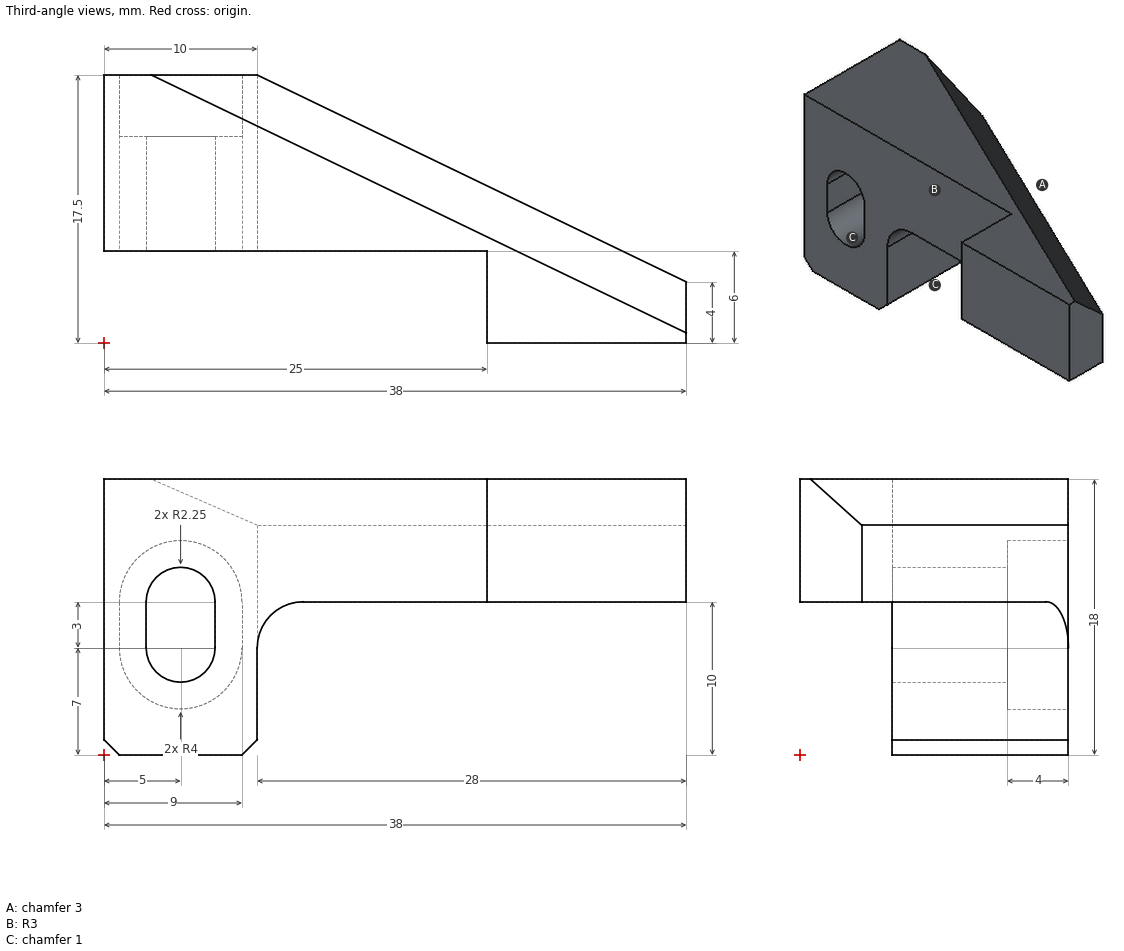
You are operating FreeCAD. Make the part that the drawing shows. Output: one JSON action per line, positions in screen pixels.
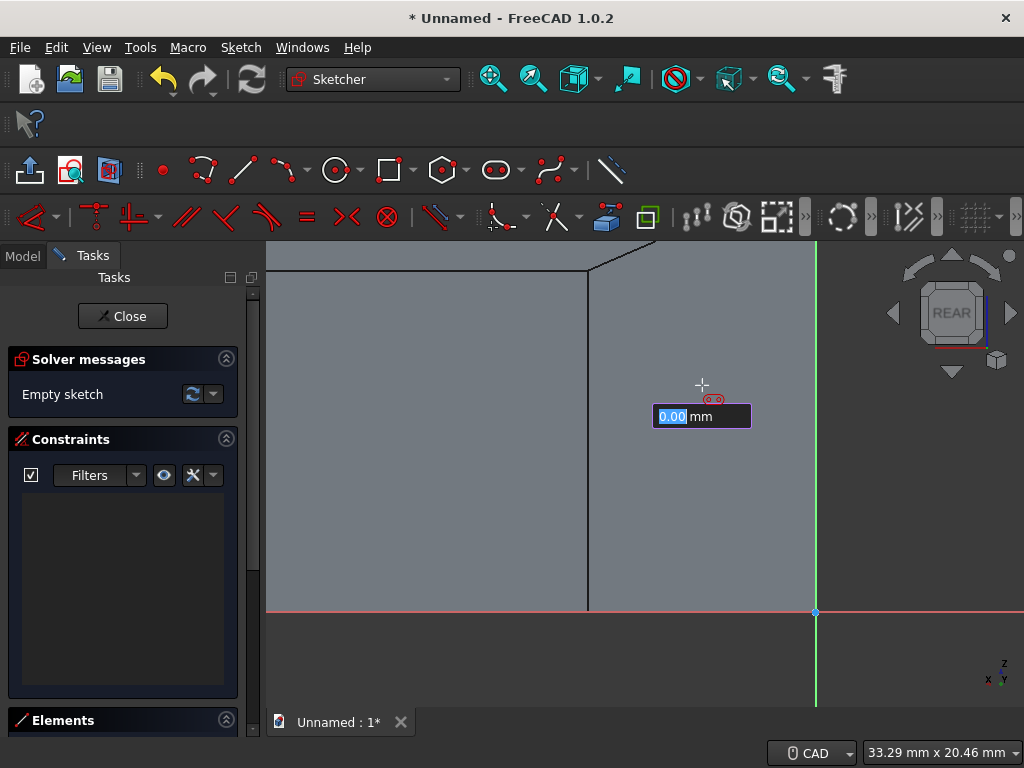
{"action": "left_click", "coordinate": [753, 419]}
{"action": "key", "text": "Escape"}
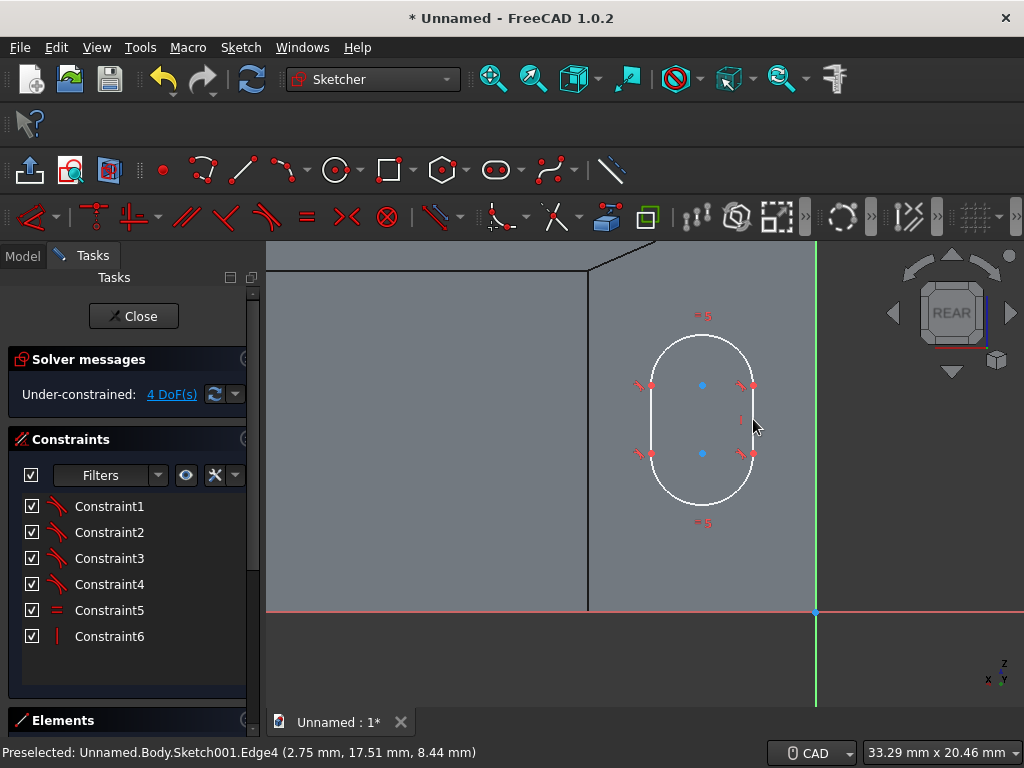
{"action": "key", "text": "d"}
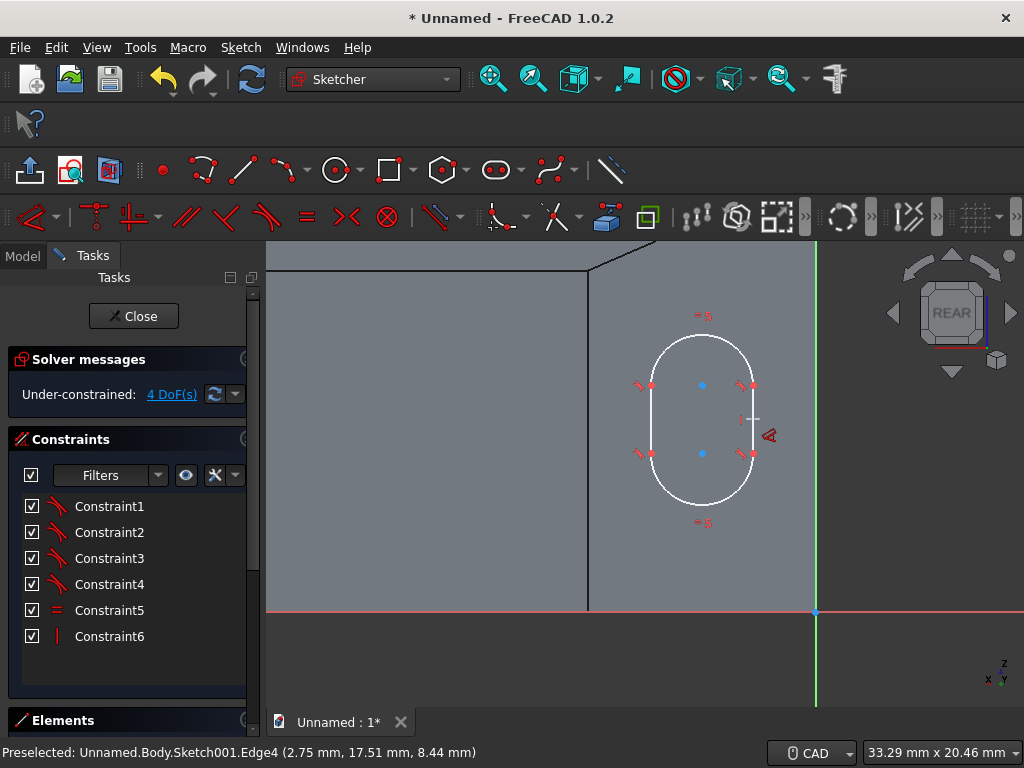
{"action": "left_click", "coordinate": [672, 495]}
{"action": "left_click", "coordinate": [653, 521]}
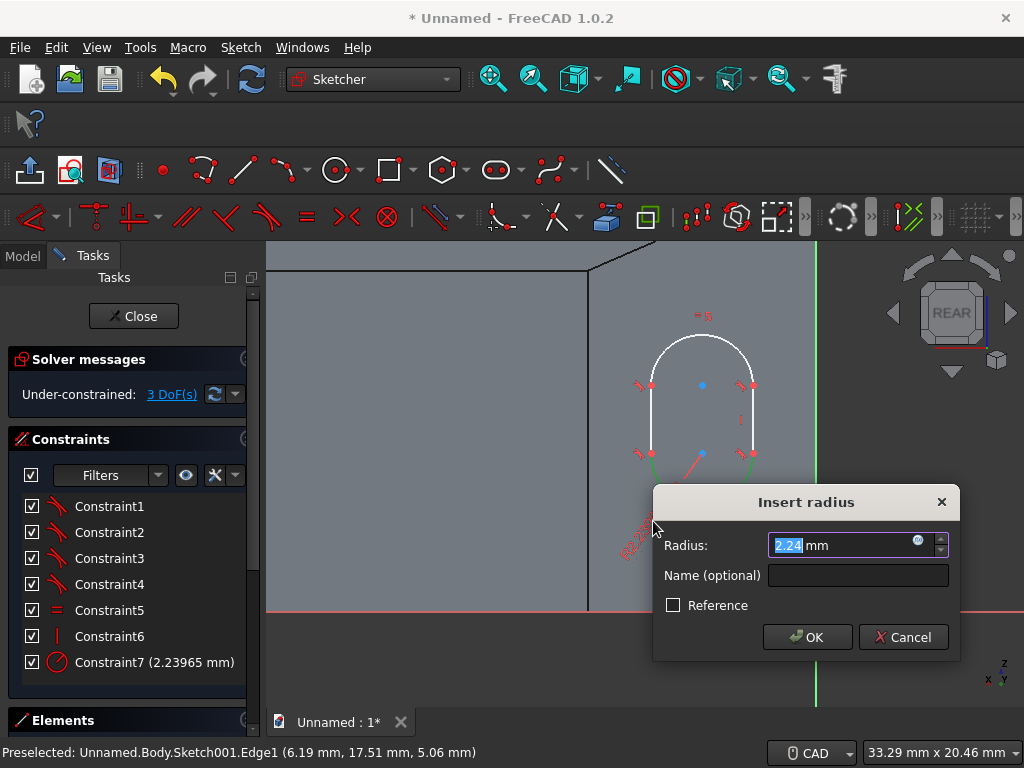
{"action": "type", "text": "2.25"}
{"action": "key", "text": "Return"}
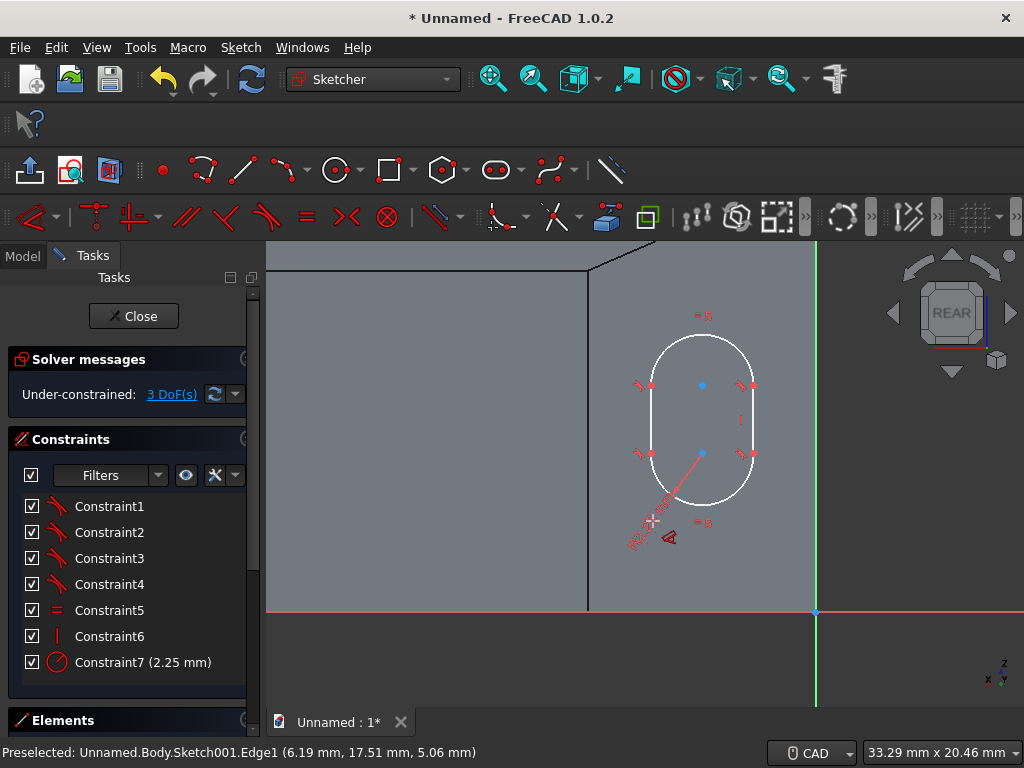
{"action": "left_click", "coordinate": [651, 434]}
{"action": "left_click", "coordinate": [617, 420]}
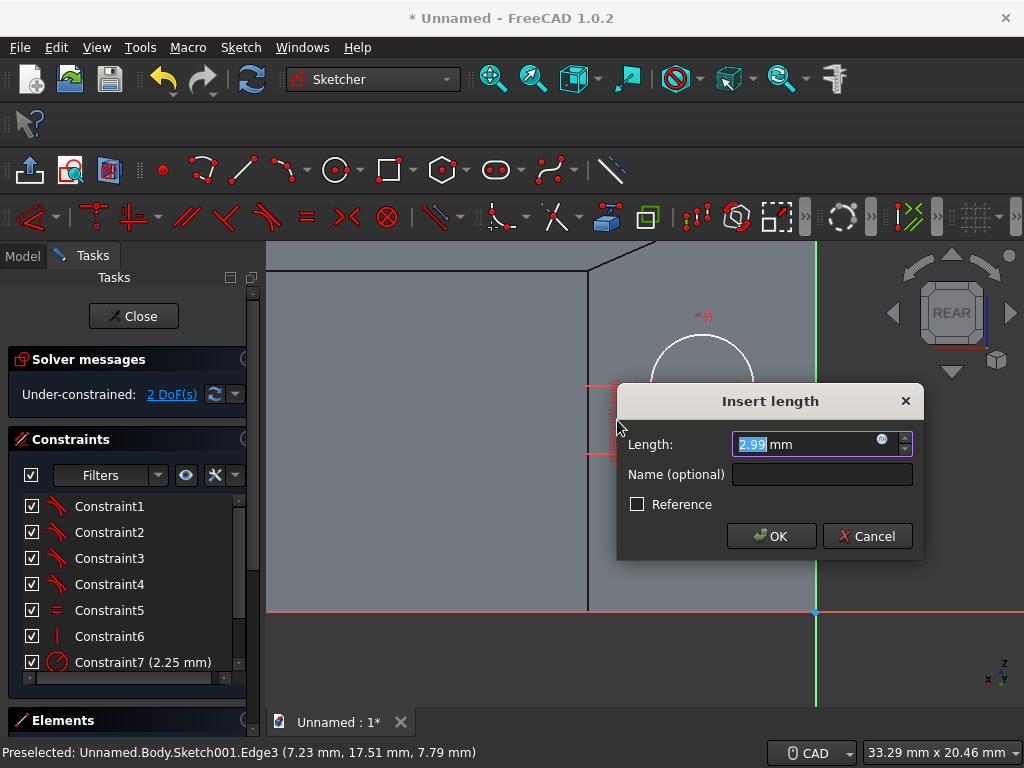
{"action": "type", "text": "3"}
{"action": "key", "text": "Return"}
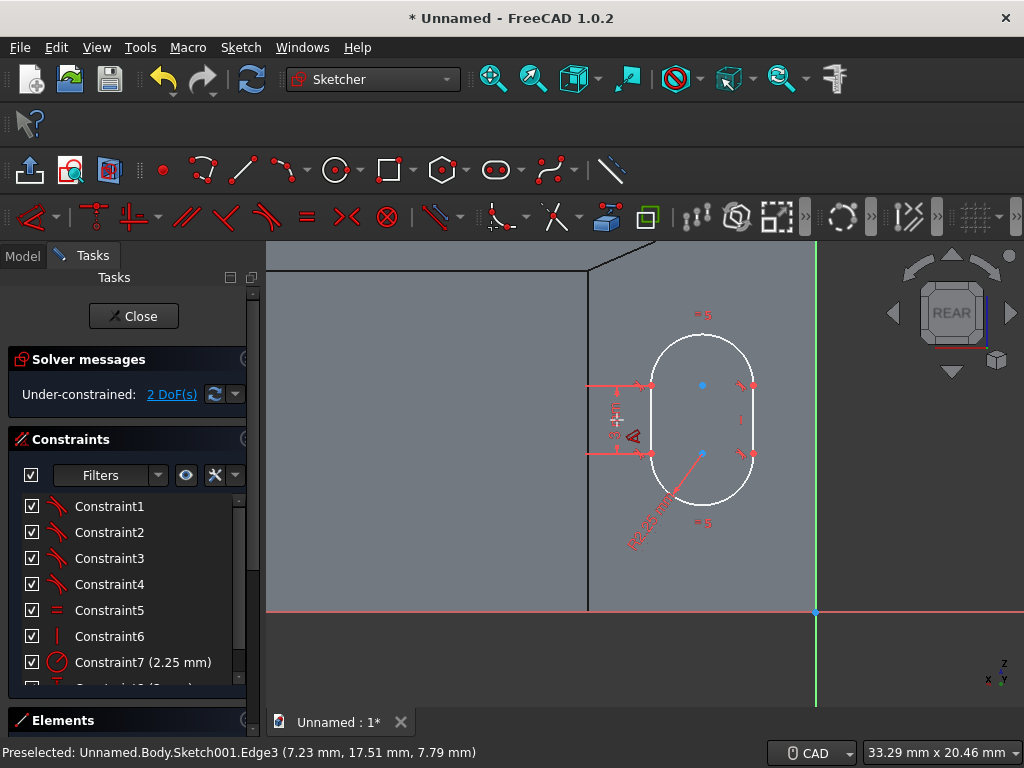
{"action": "left_click", "coordinate": [651, 454]}
{"action": "left_click", "coordinate": [850, 533]}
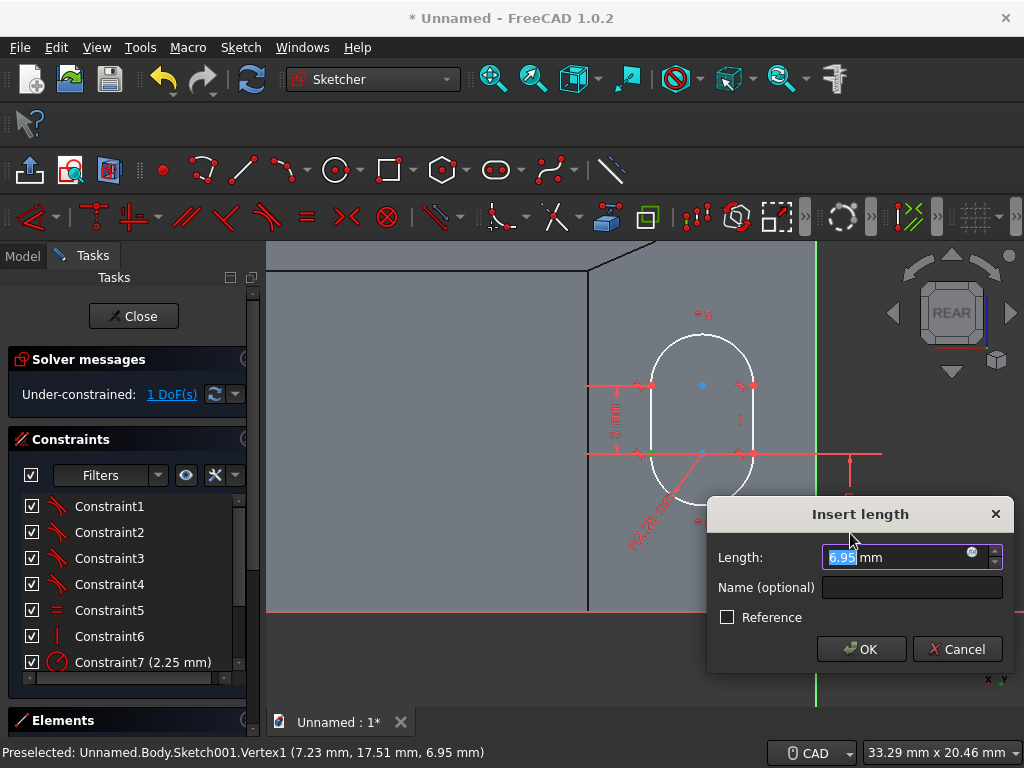
{"action": "type", "text": "7"}
{"action": "key", "text": "Return"}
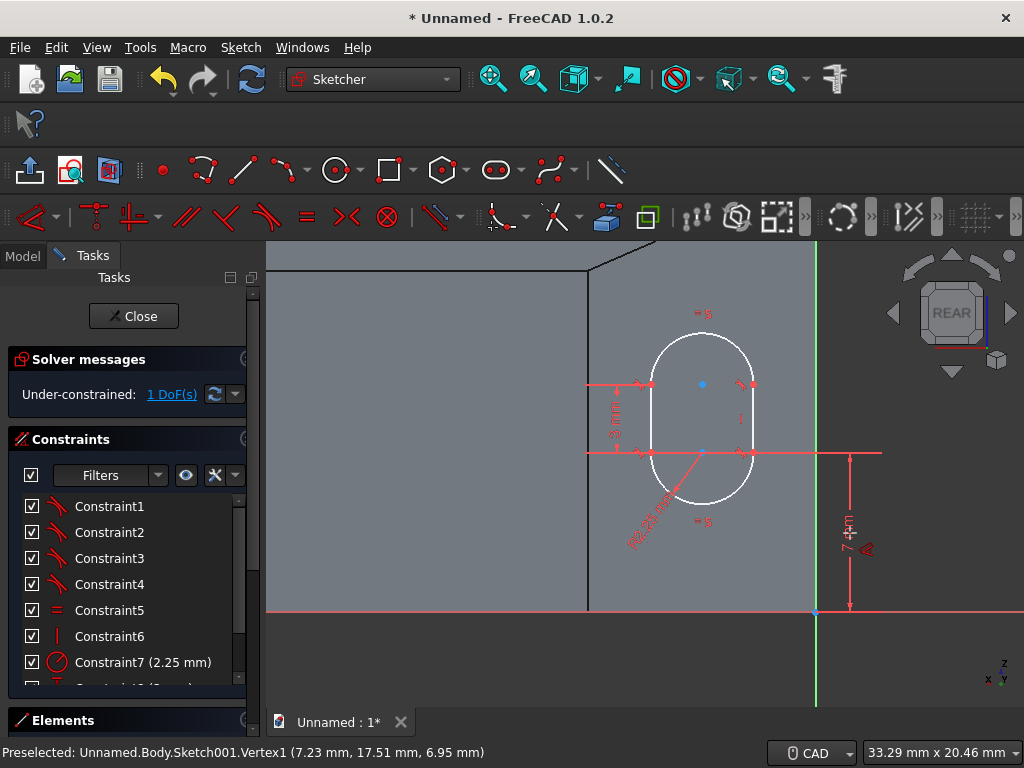
{"action": "left_click", "coordinate": [702, 453]}
{"action": "left_click", "coordinate": [759, 646]}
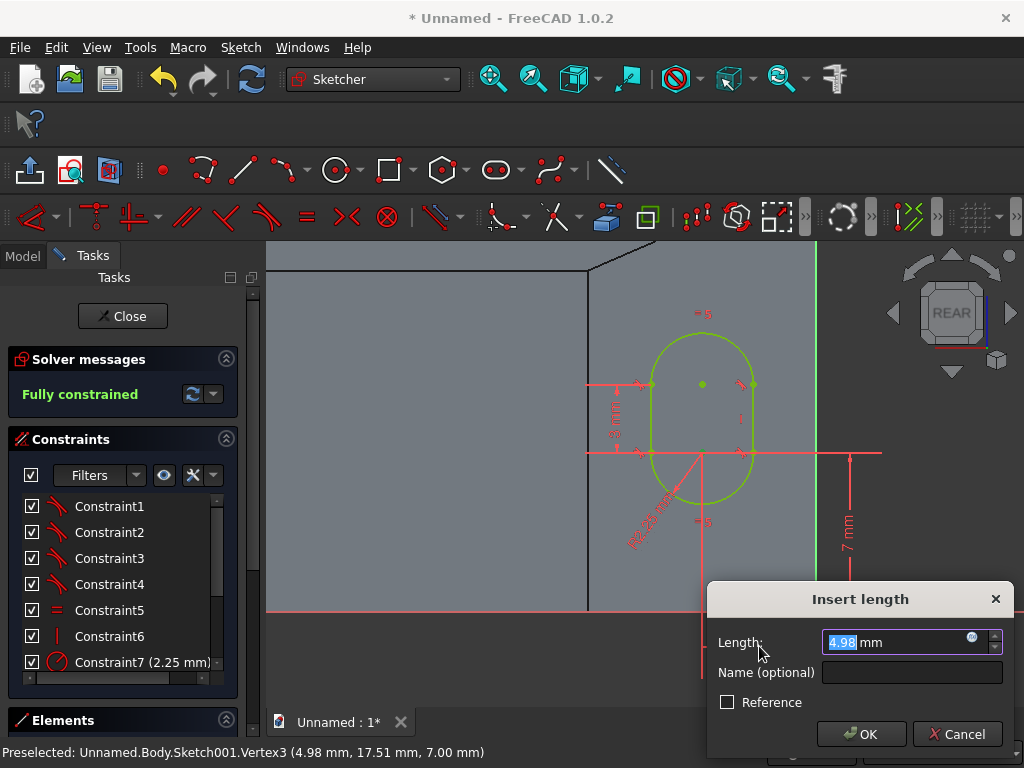
{"action": "type", "text": "5"}
{"action": "key", "text": "Return"}
{"action": "key", "text": "Escape"}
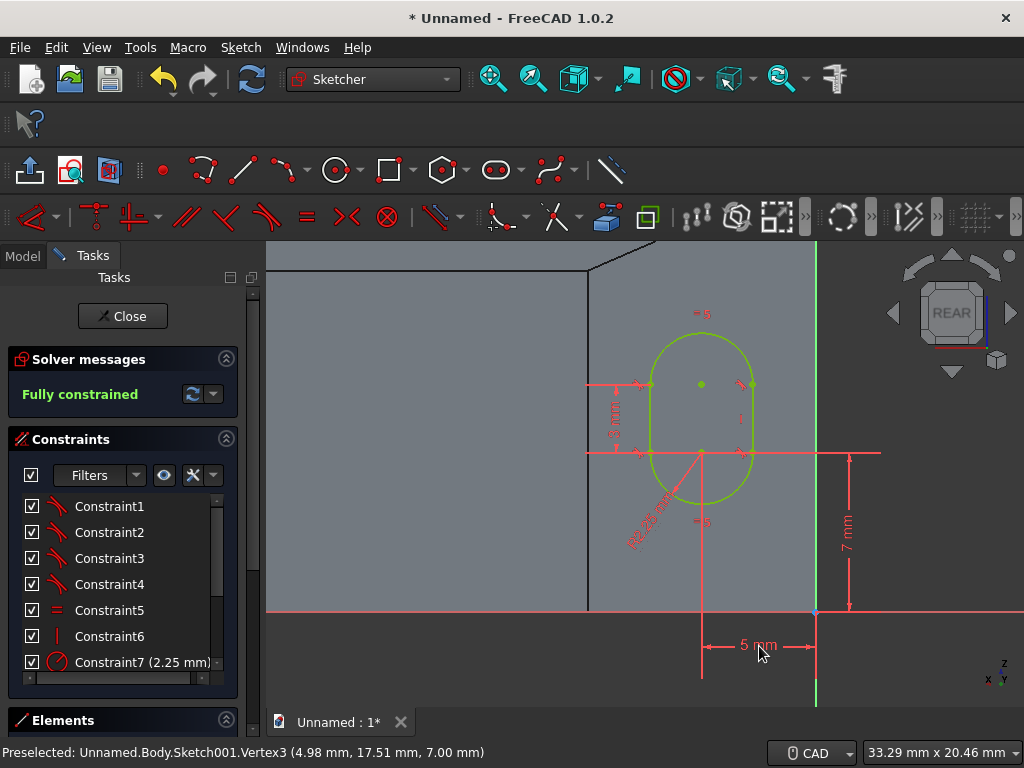
{"action": "left_click", "coordinate": [123, 316]}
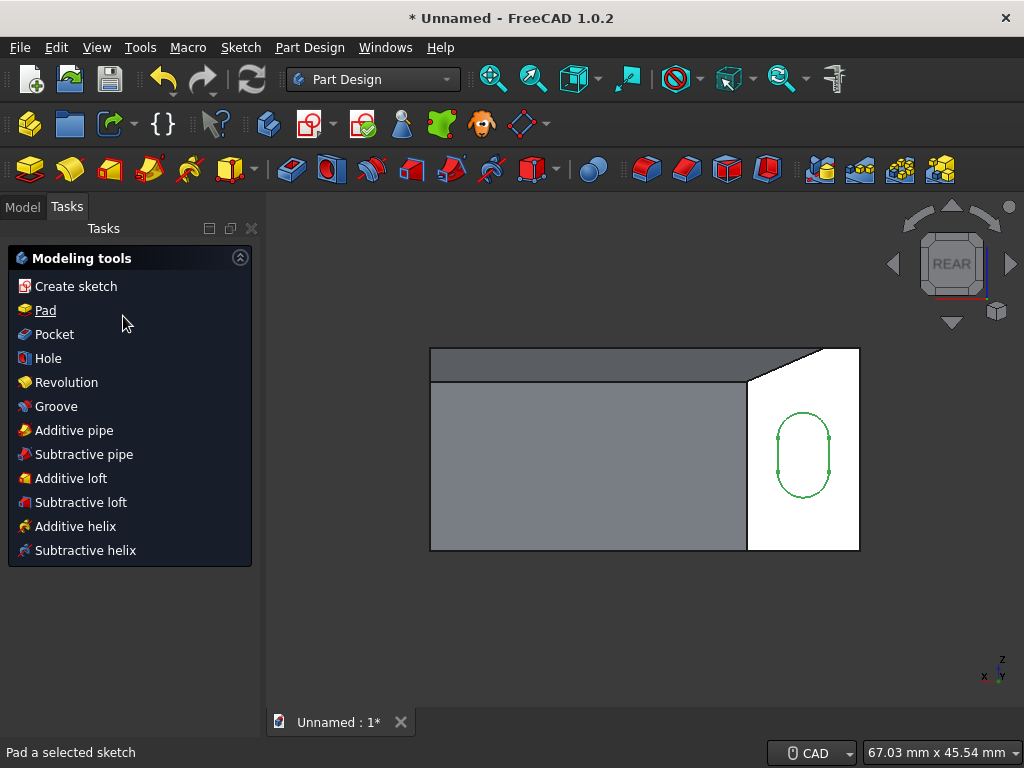
{"action": "left_click", "coordinate": [292, 170]}